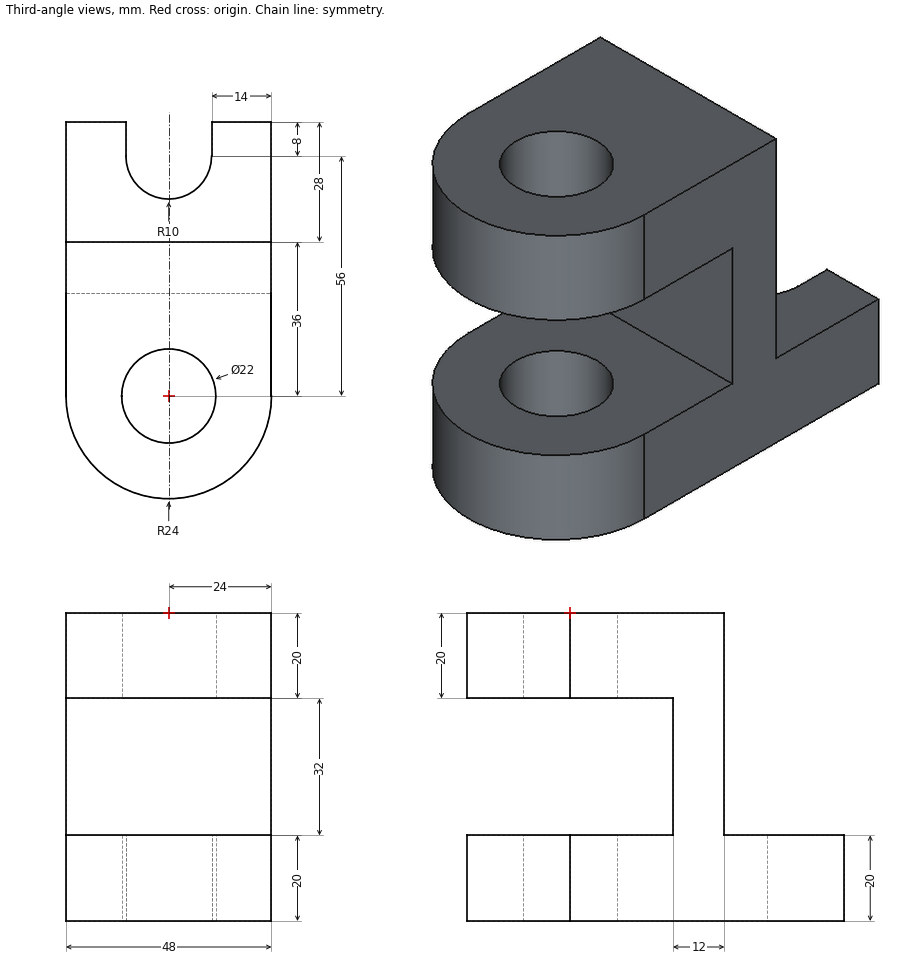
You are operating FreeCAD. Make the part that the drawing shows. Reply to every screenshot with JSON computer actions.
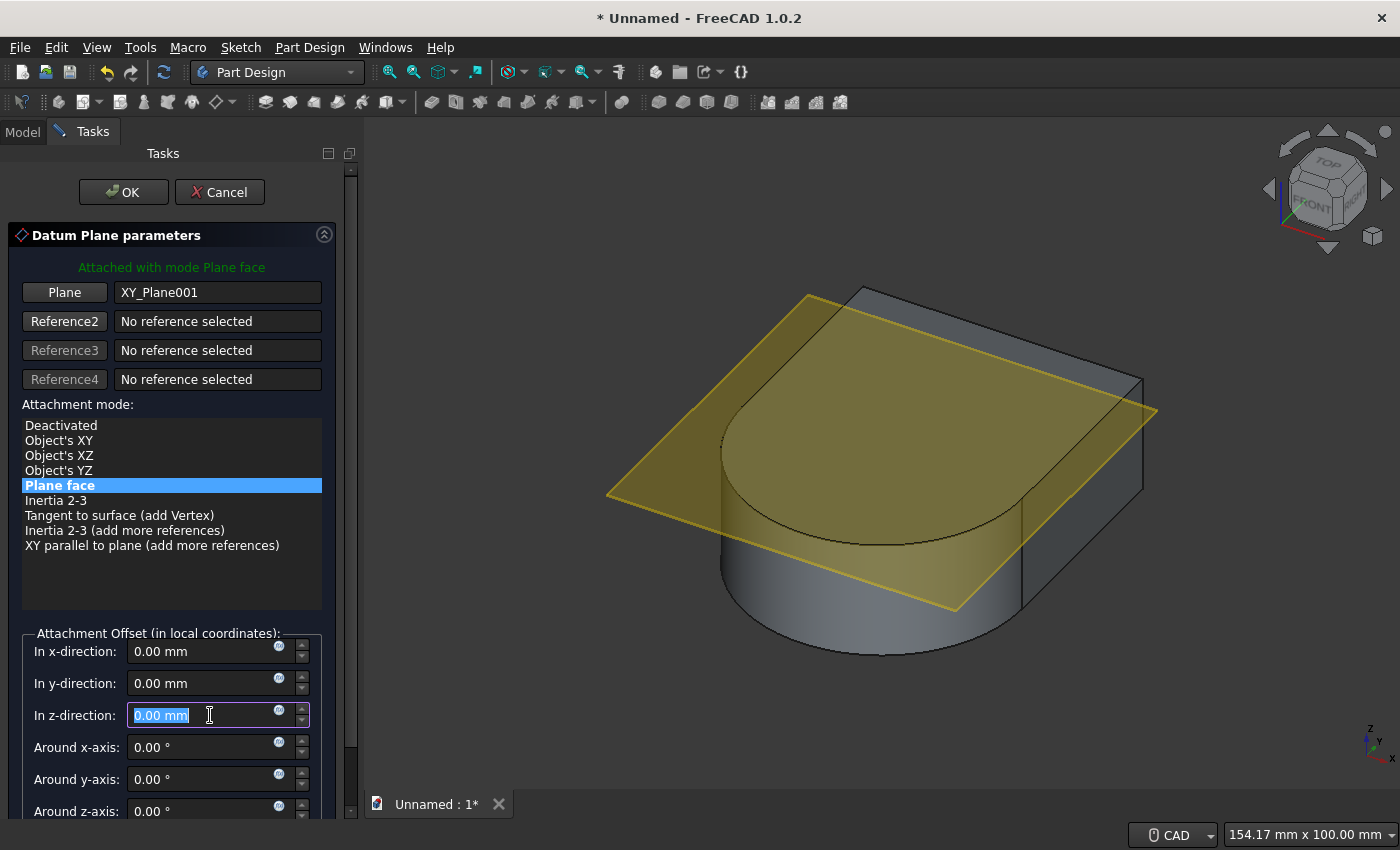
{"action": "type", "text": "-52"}
{"action": "key", "text": "Tab"}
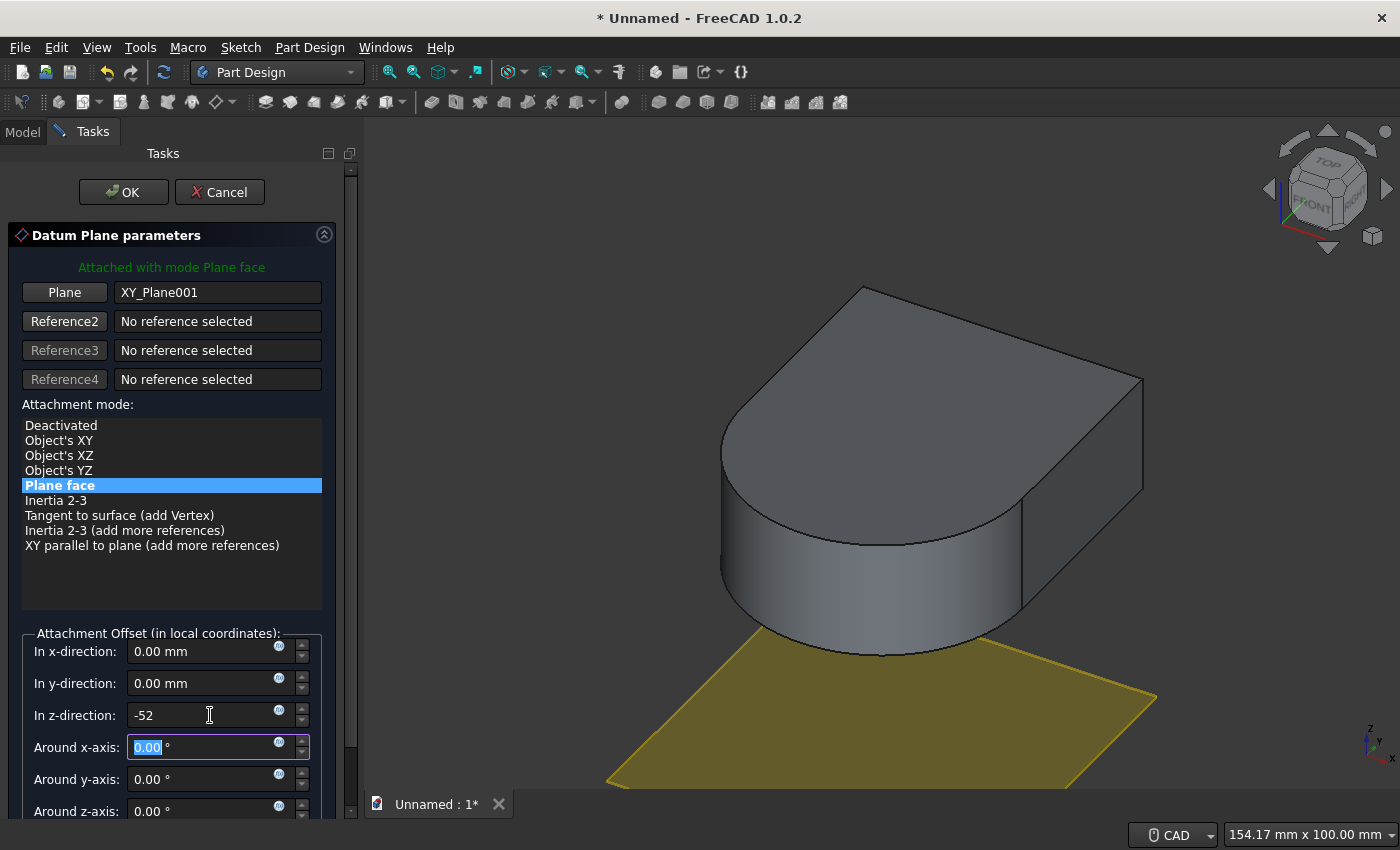
{"action": "left_click", "coordinate": [124, 192]}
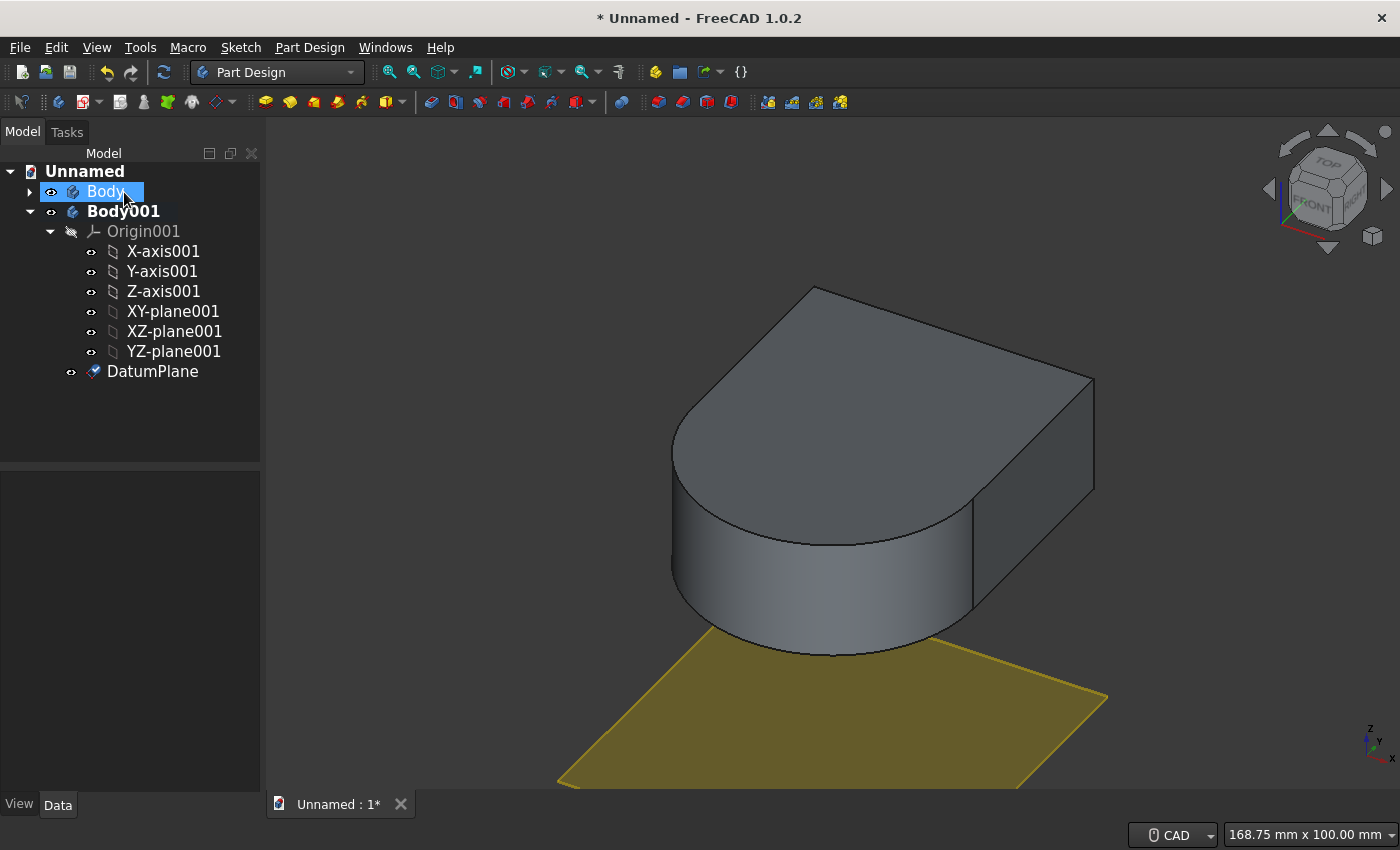
{"action": "left_click", "coordinate": [116, 372]}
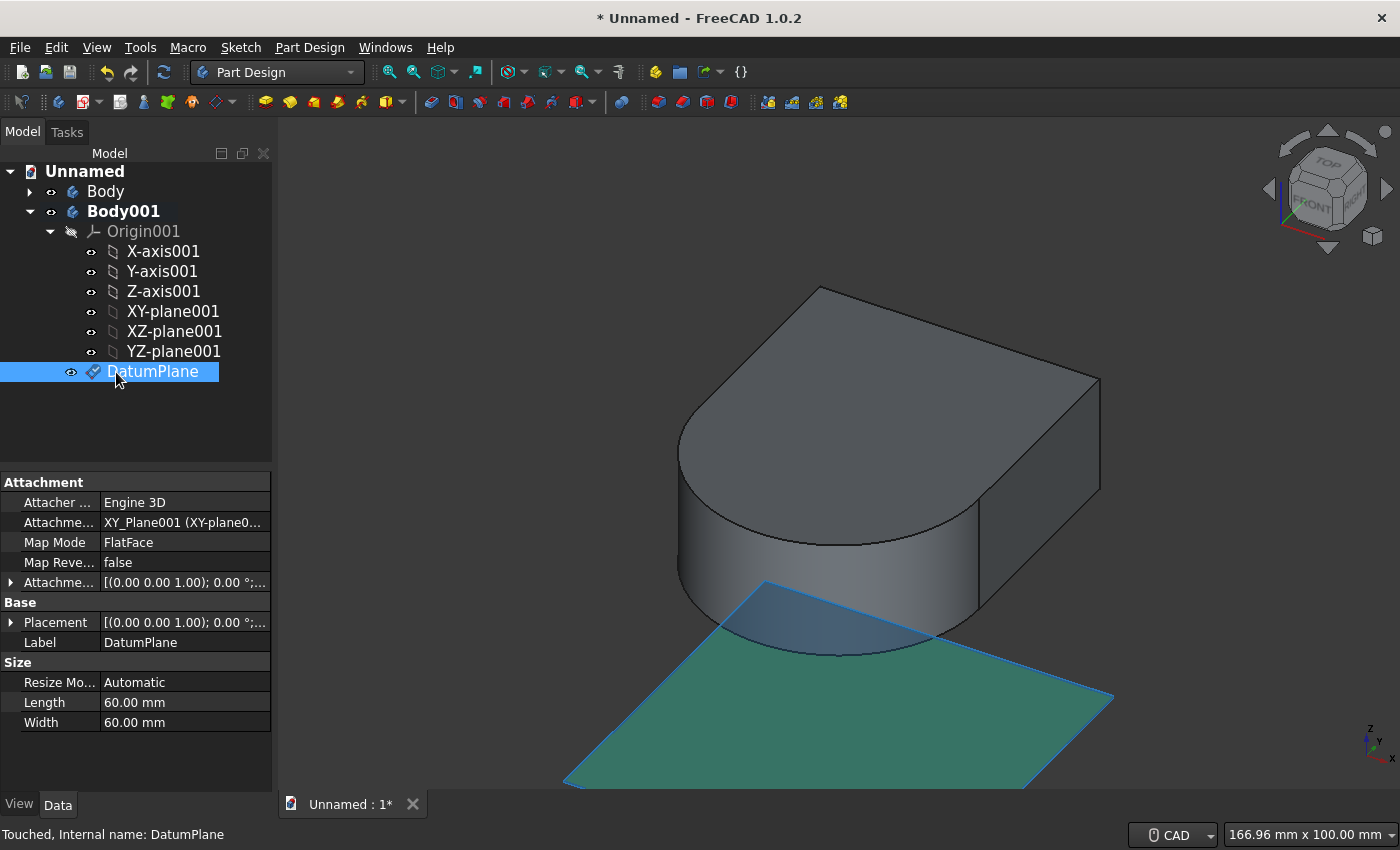
{"action": "left_click", "coordinate": [84, 102]}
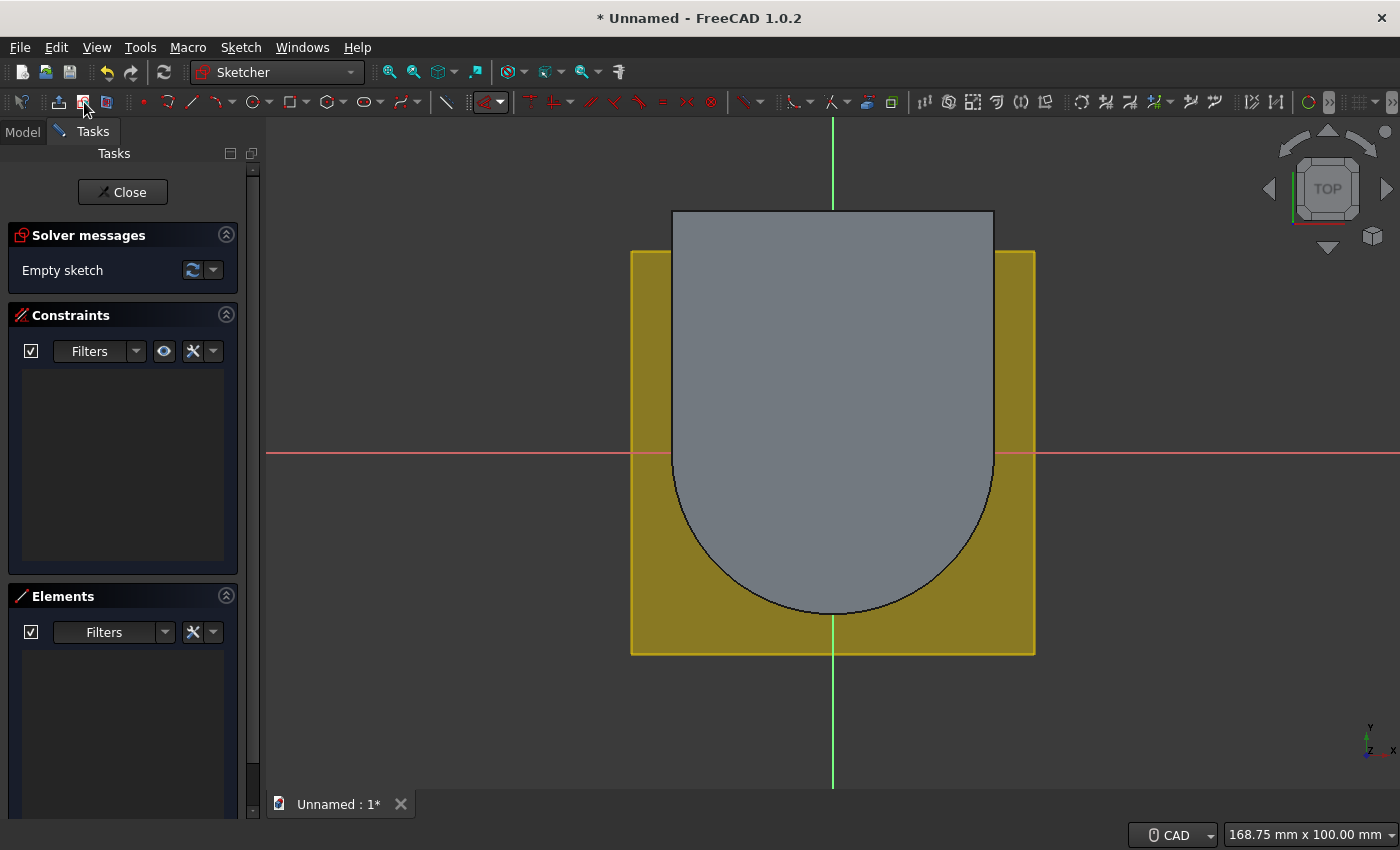
{"action": "key", "text": "g m"}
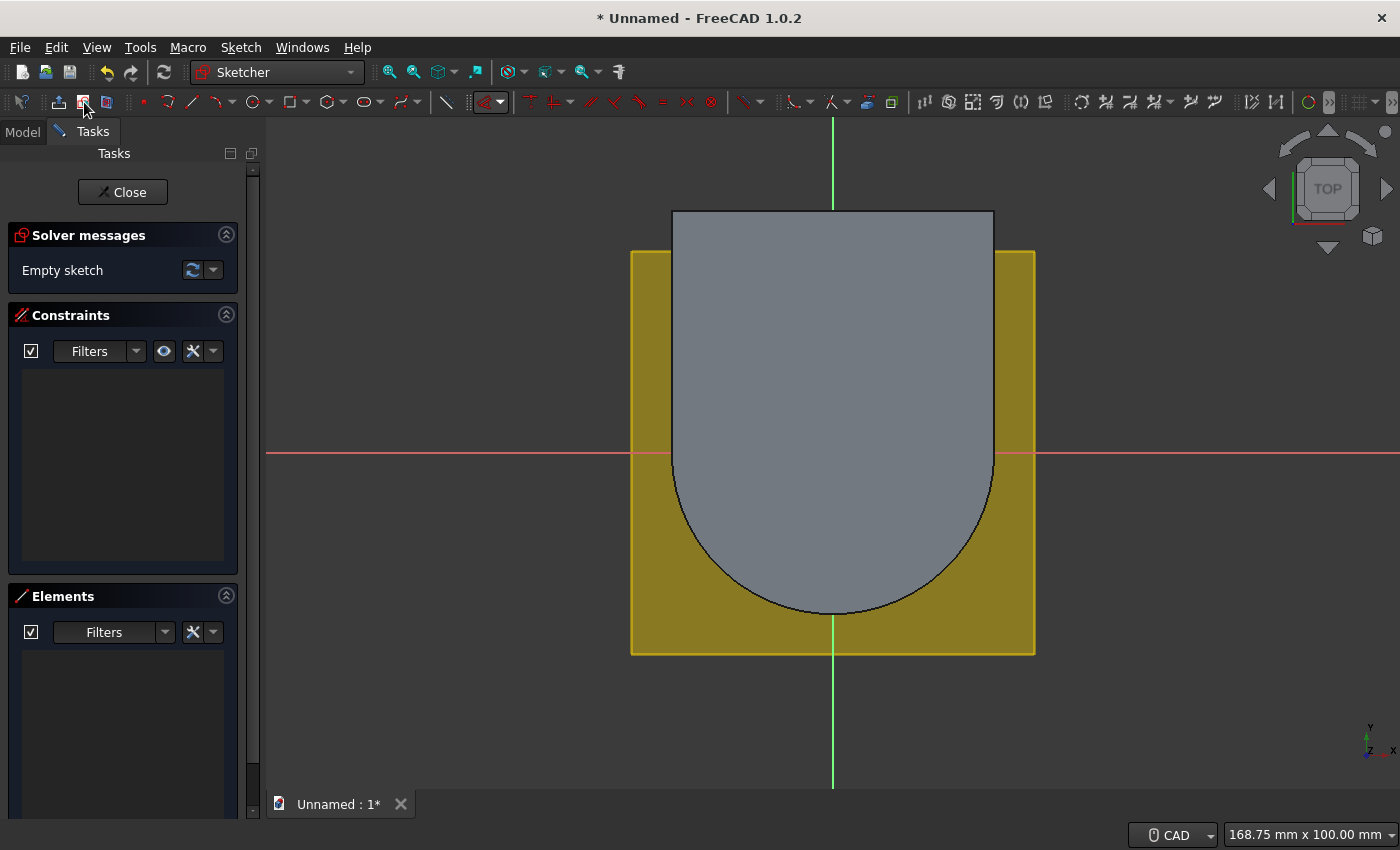
{"action": "left_click", "coordinate": [672, 453]}
{"action": "left_click", "coordinate": [672, 211]}
{"action": "left_click", "coordinate": [994, 211]}
{"action": "left_click", "coordinate": [994, 453]}
{"action": "right_click", "coordinate": [994, 453]}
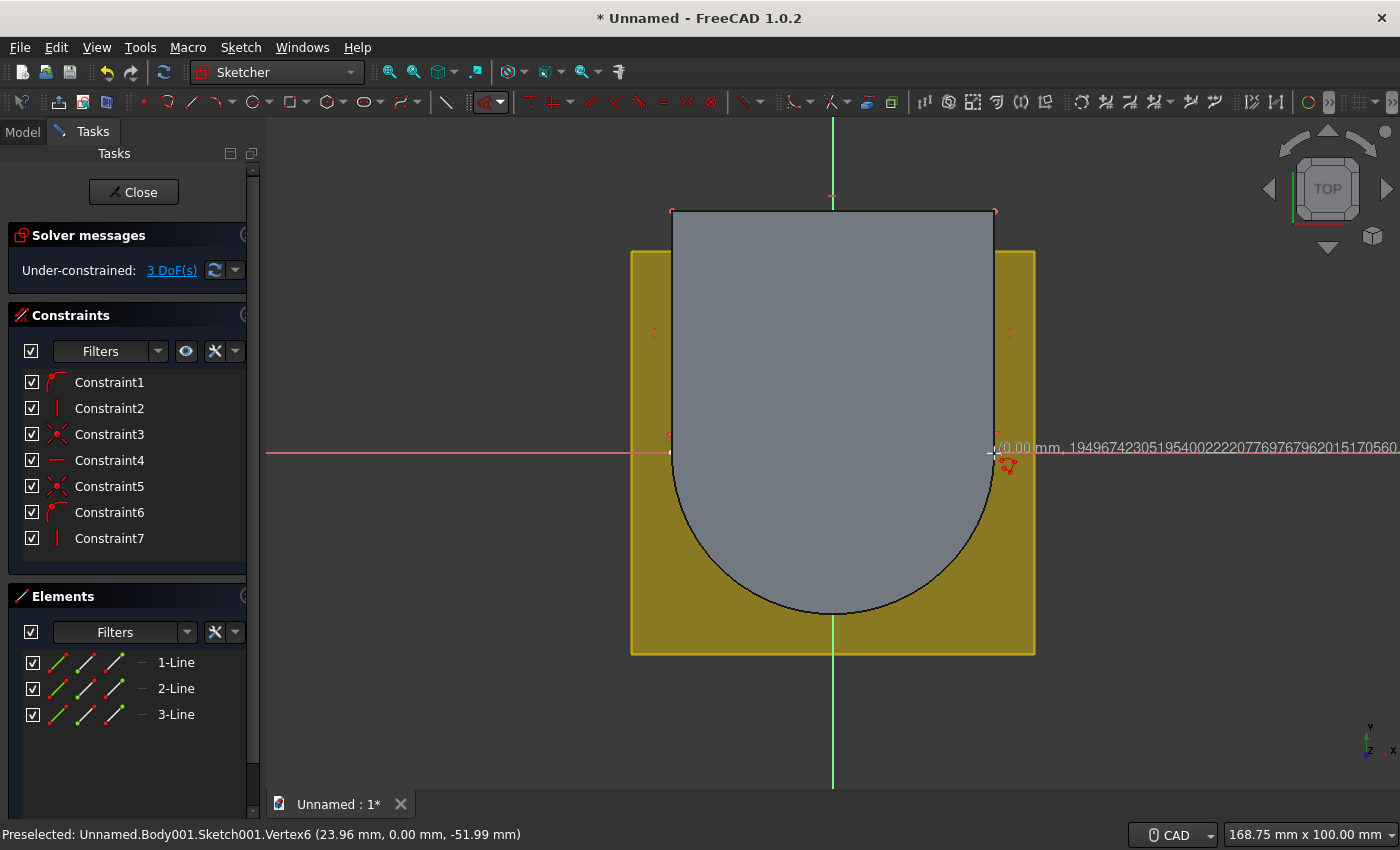
{"action": "key", "text": "g 3 a"}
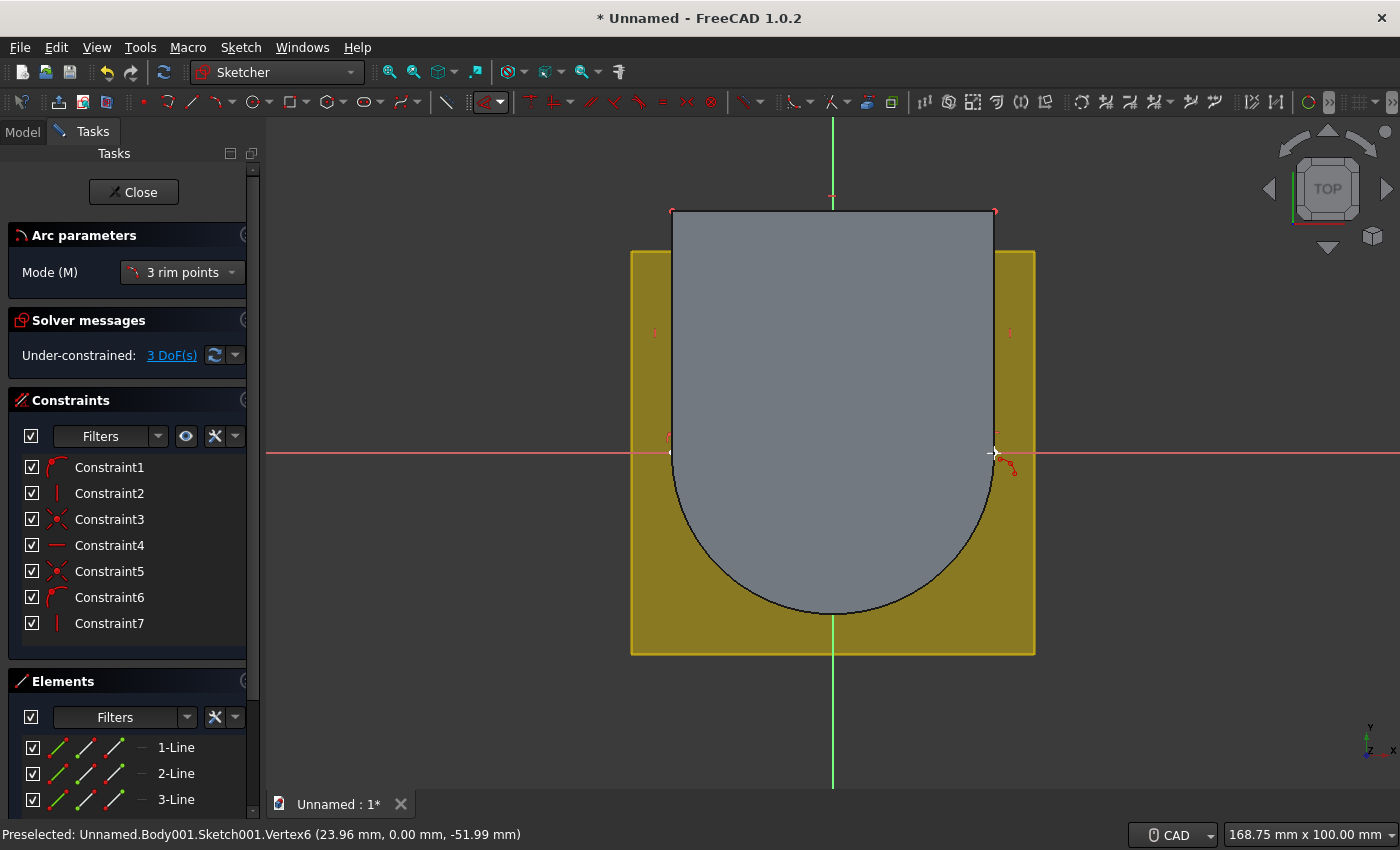
{"action": "left_click", "coordinate": [994, 453]}
{"action": "left_click", "coordinate": [672, 453]}
{"action": "left_click", "coordinate": [783, 606]}
{"action": "key", "text": "Escape"}